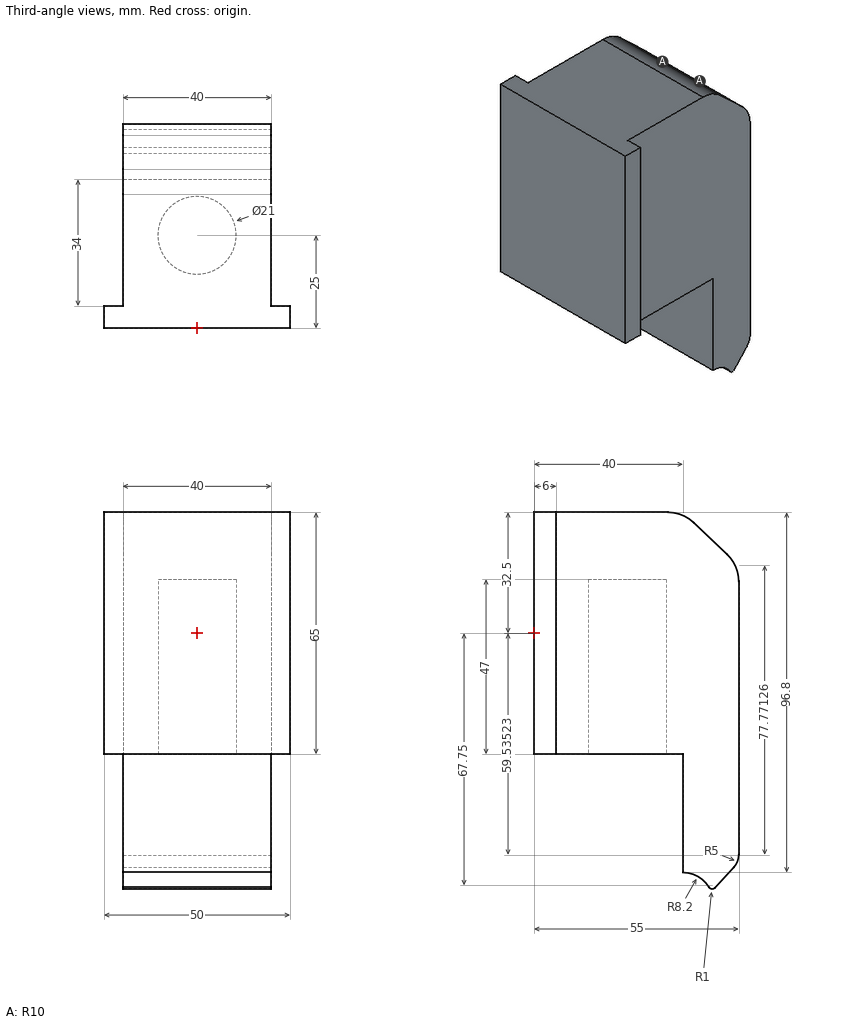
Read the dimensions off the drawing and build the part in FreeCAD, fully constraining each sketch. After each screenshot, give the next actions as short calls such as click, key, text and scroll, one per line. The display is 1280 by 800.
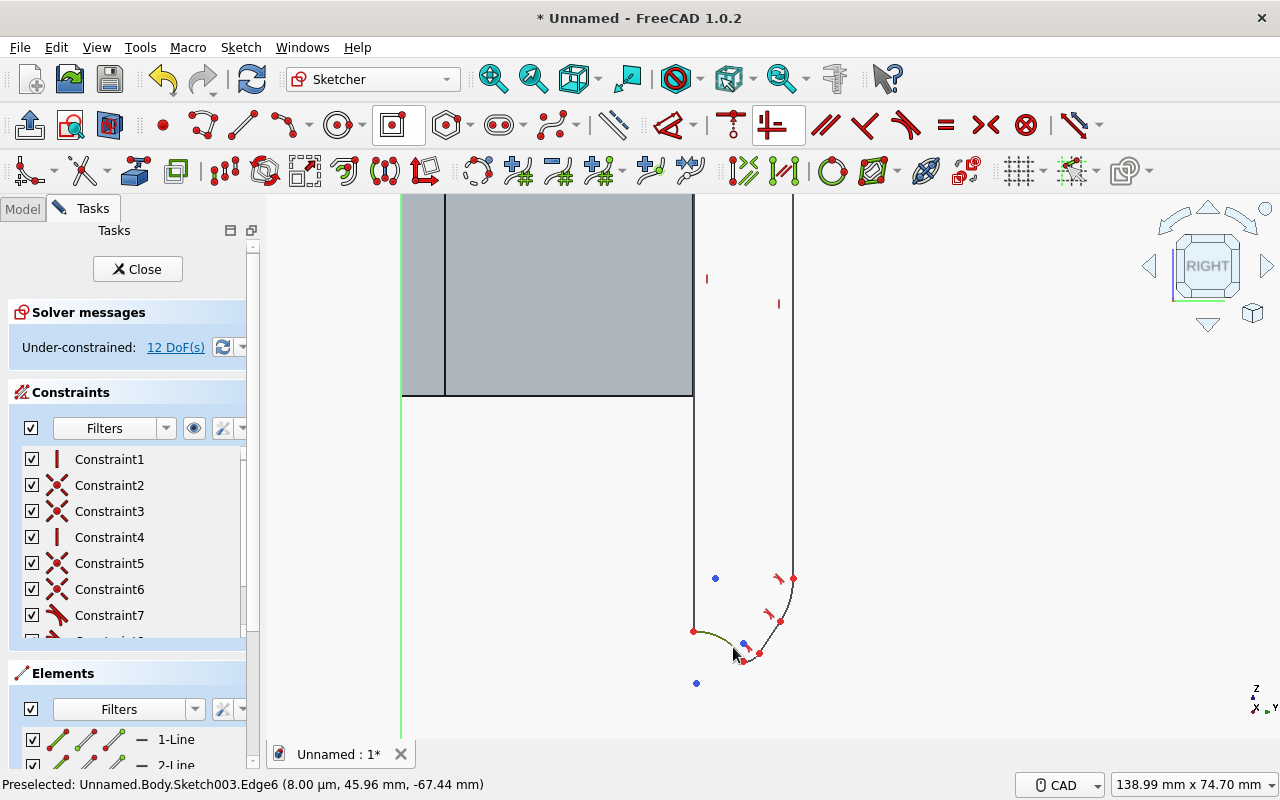
scroll(752, 660, up, 3)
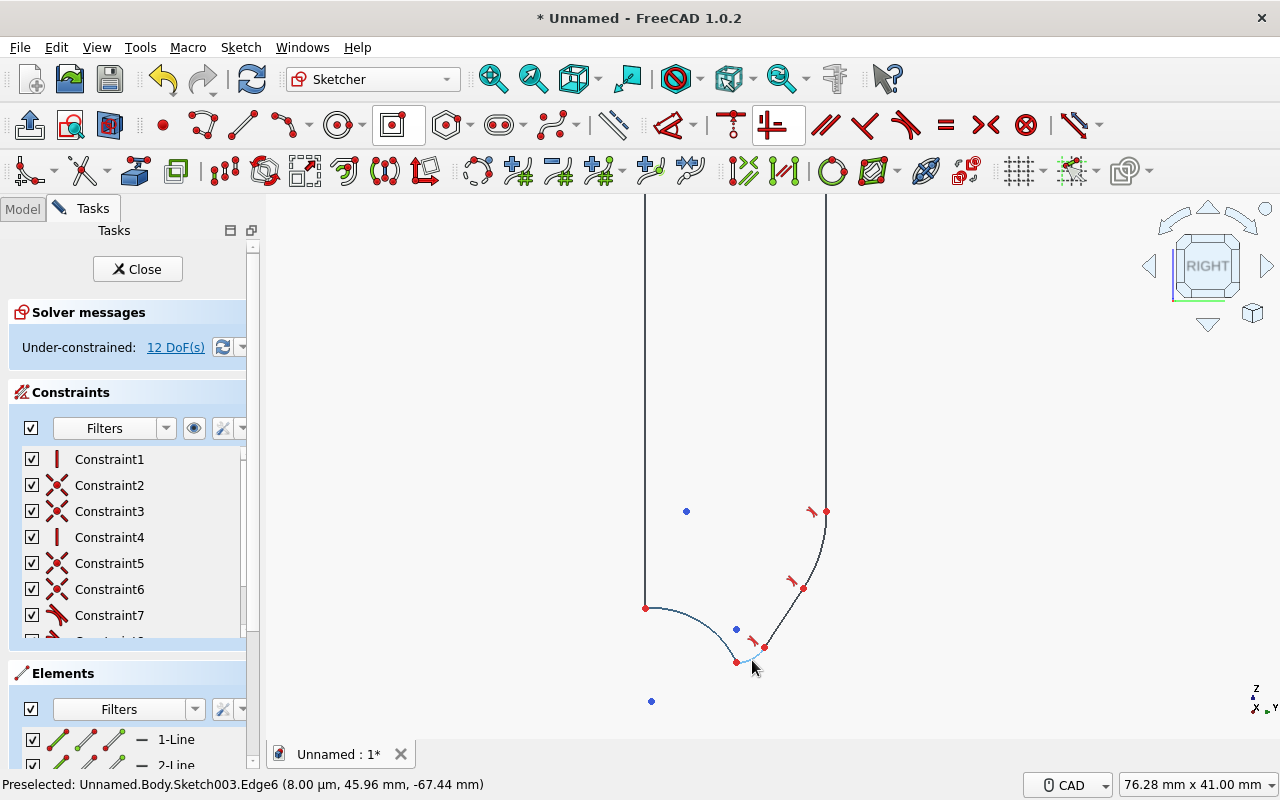
click(752, 659)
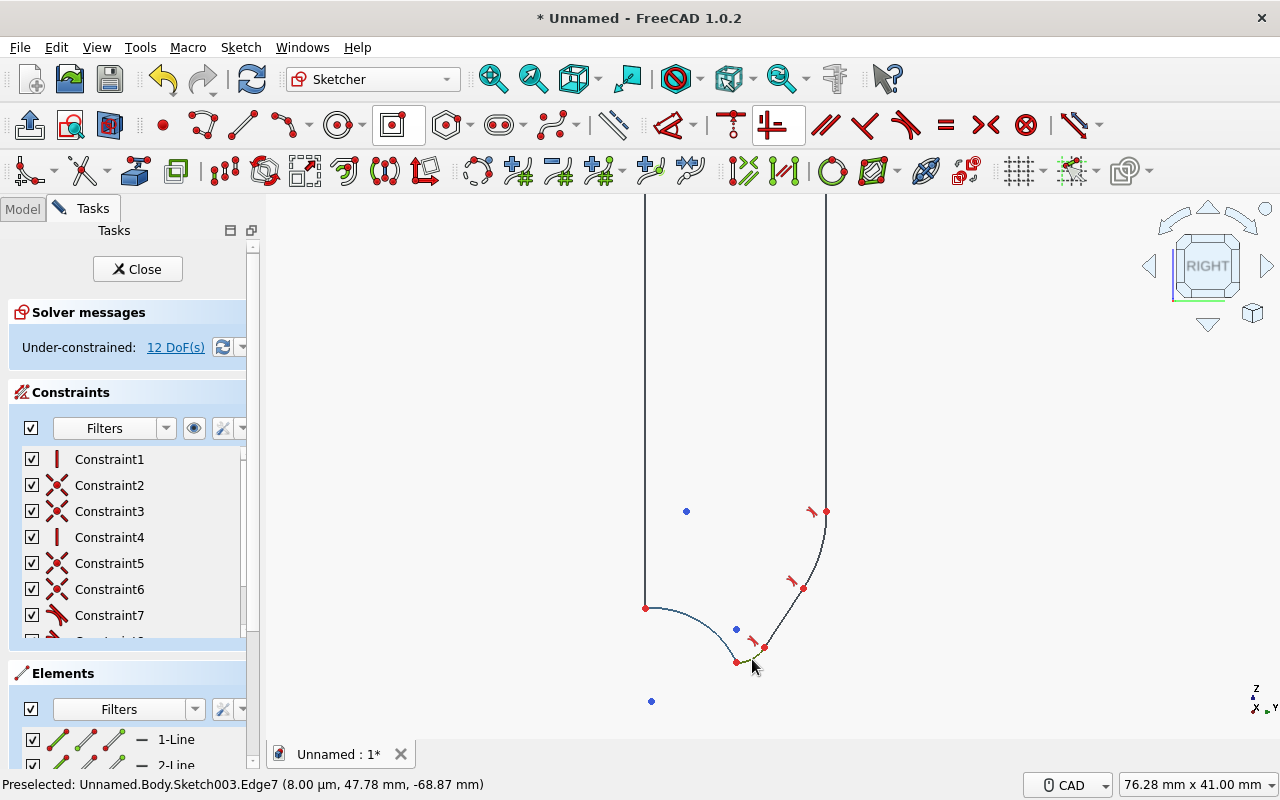
key(t)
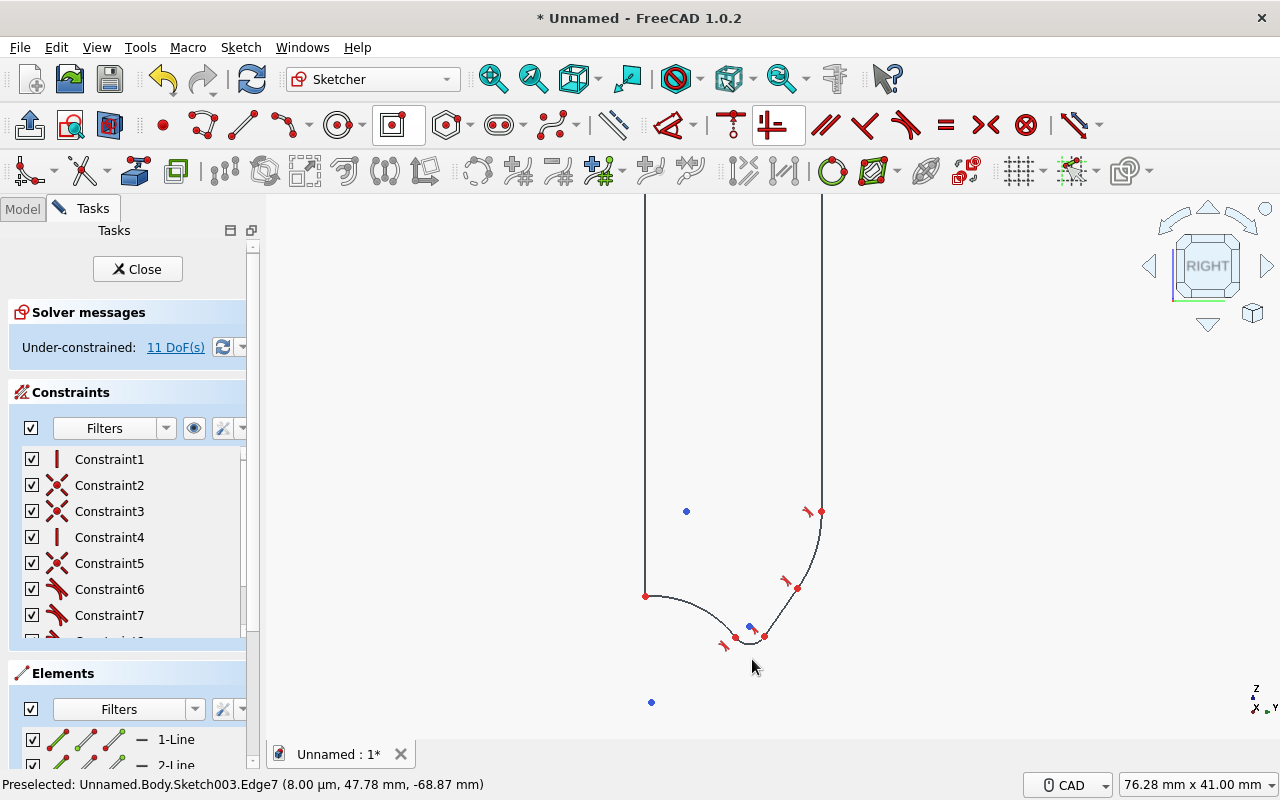
click(668, 126)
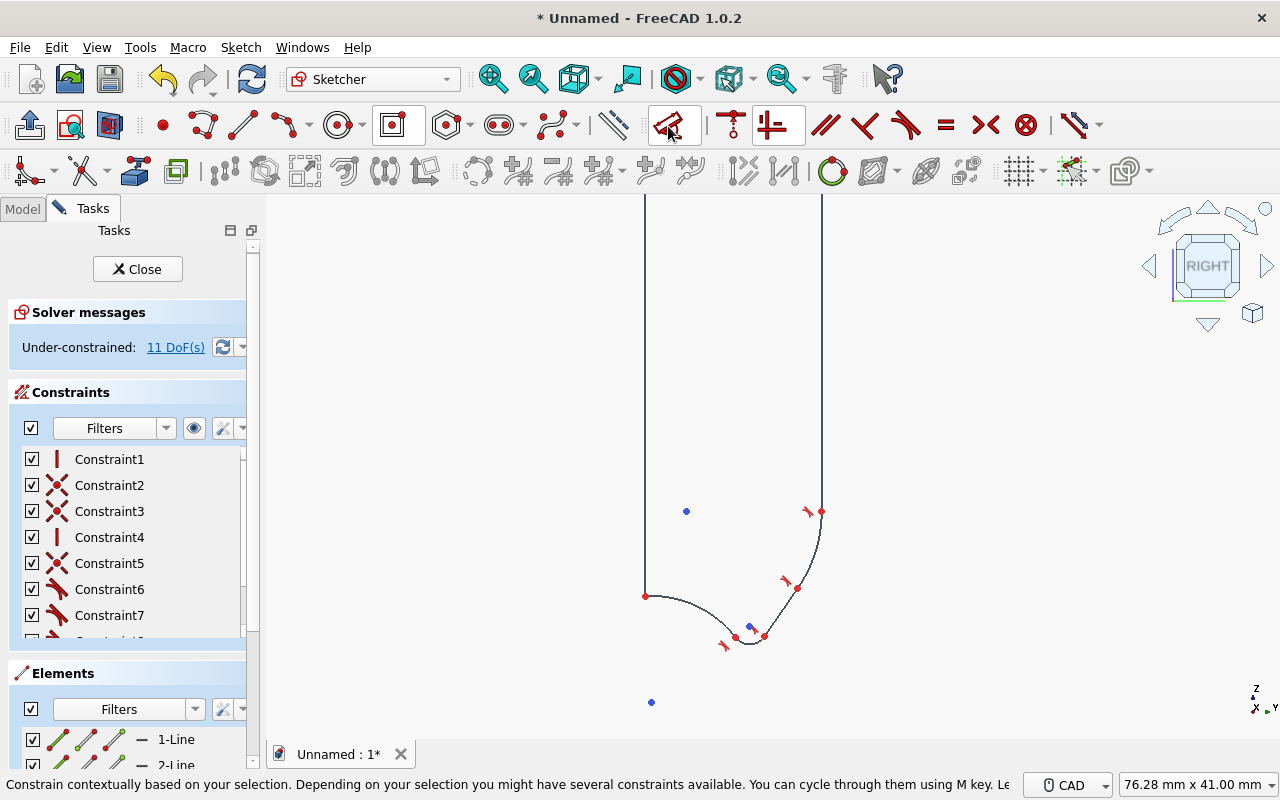
click(810, 567)
click(839, 580)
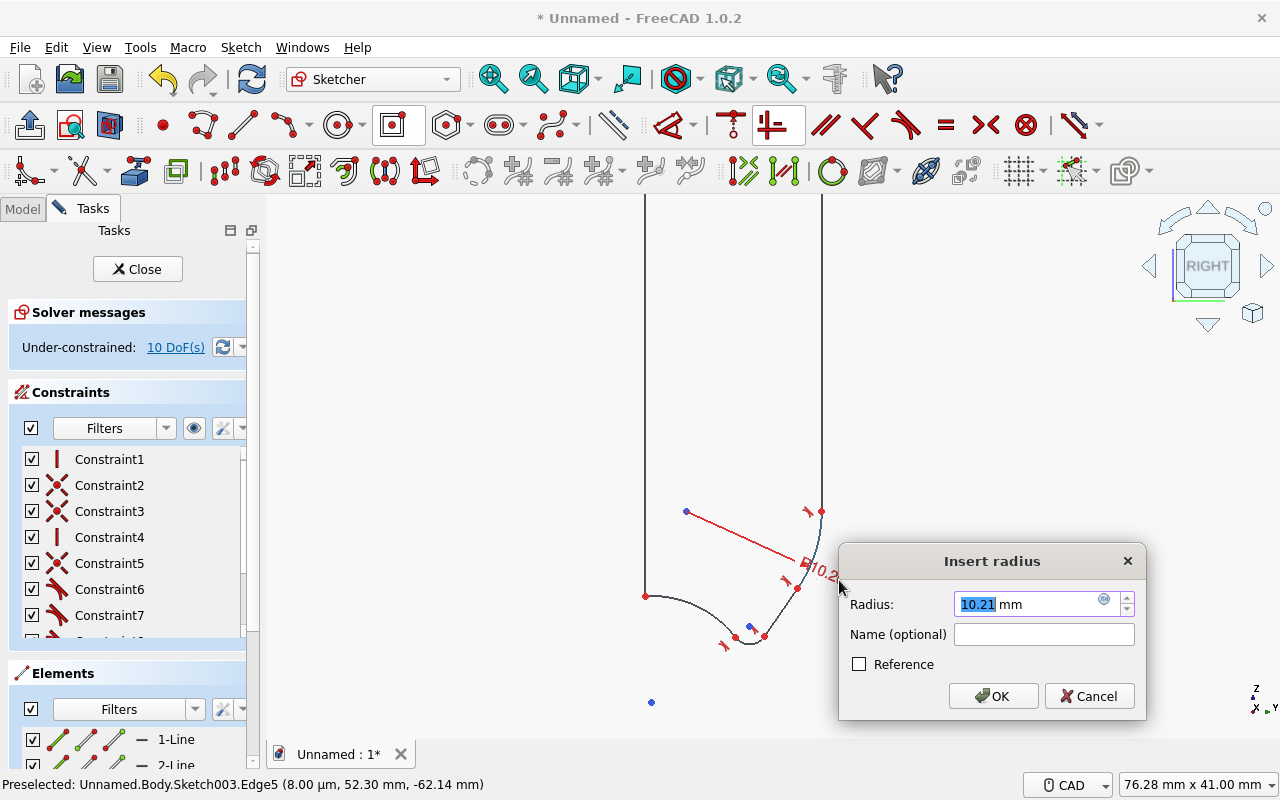
text(5)
key(Return)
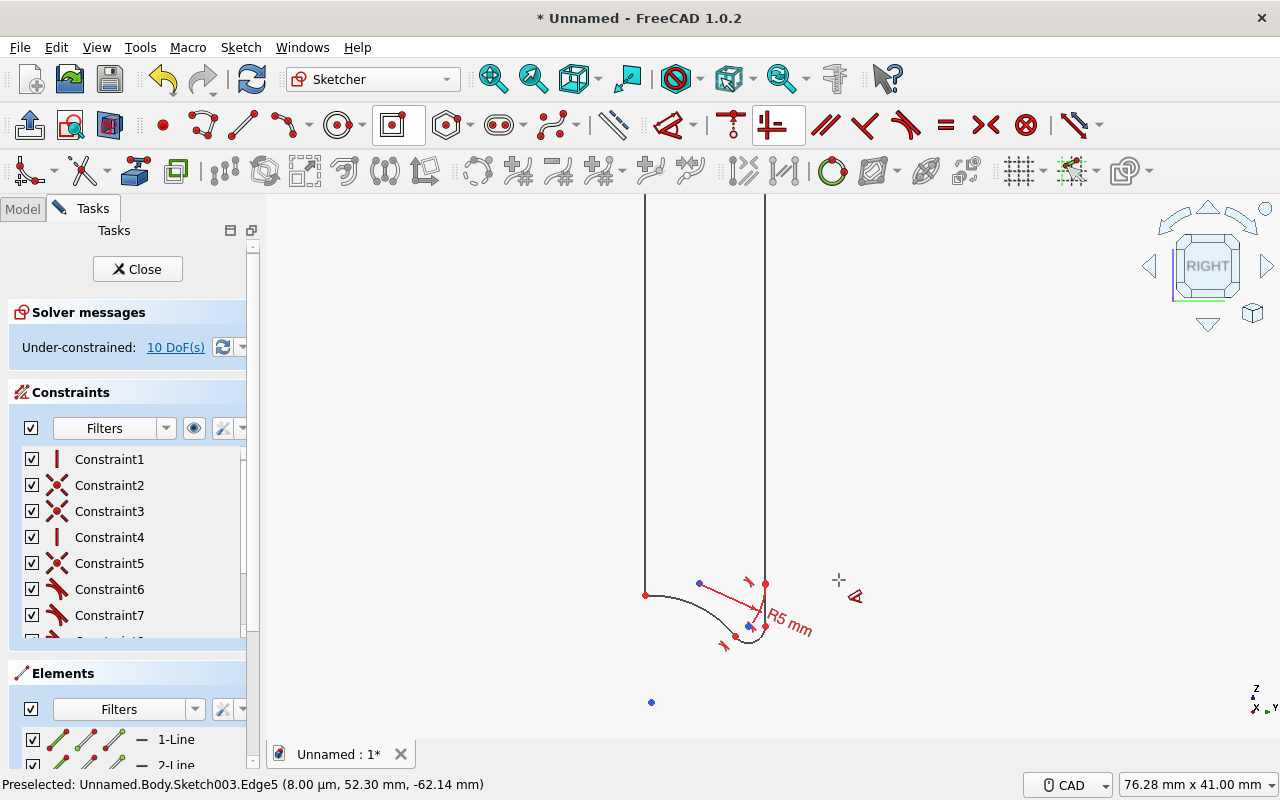
click(713, 615)
click(731, 589)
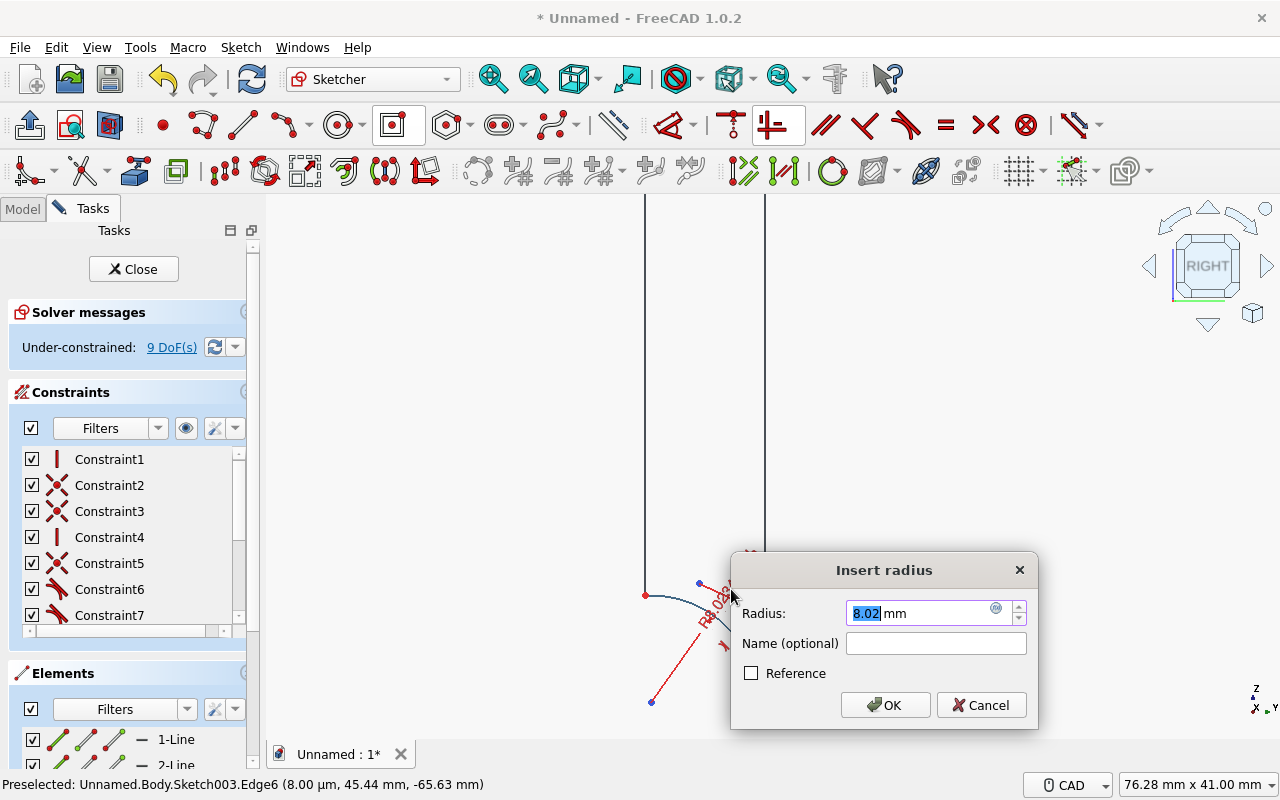
text(8.2)
key(Return)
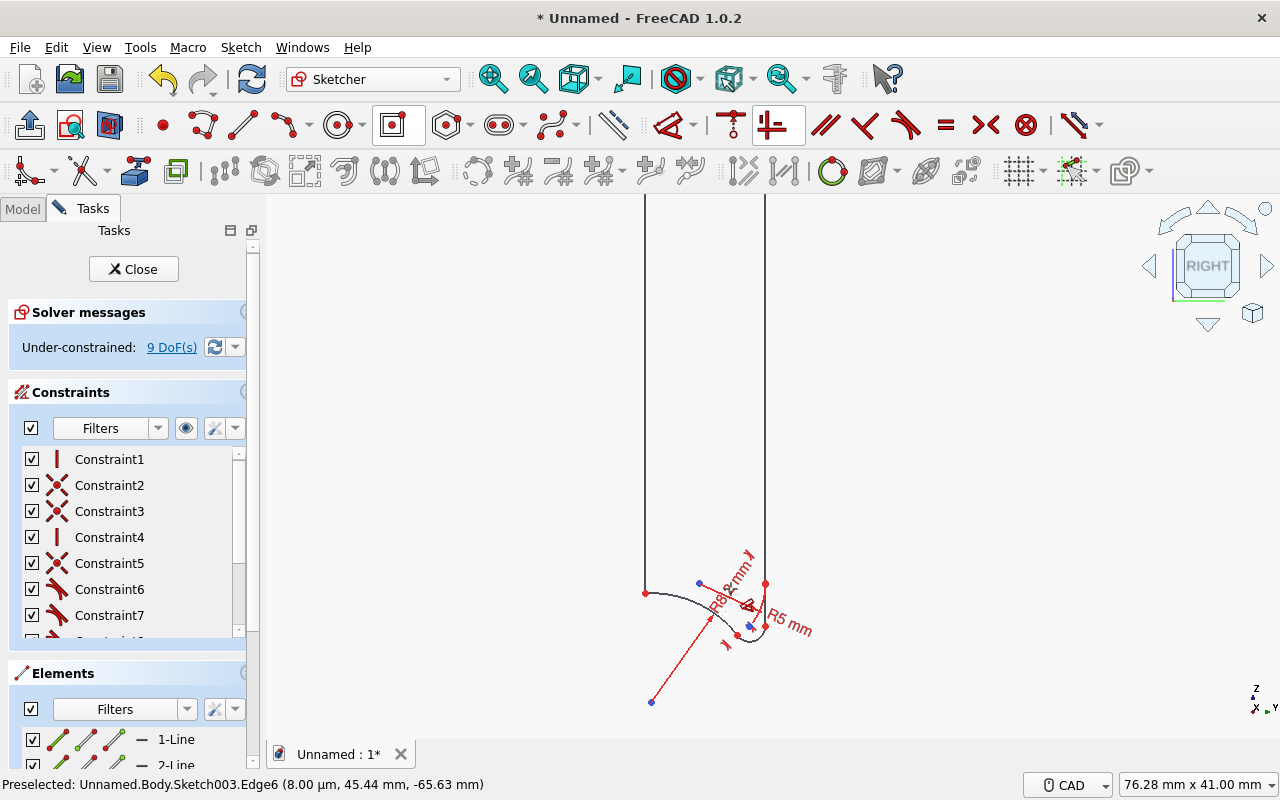
scroll(747, 642, up, 6)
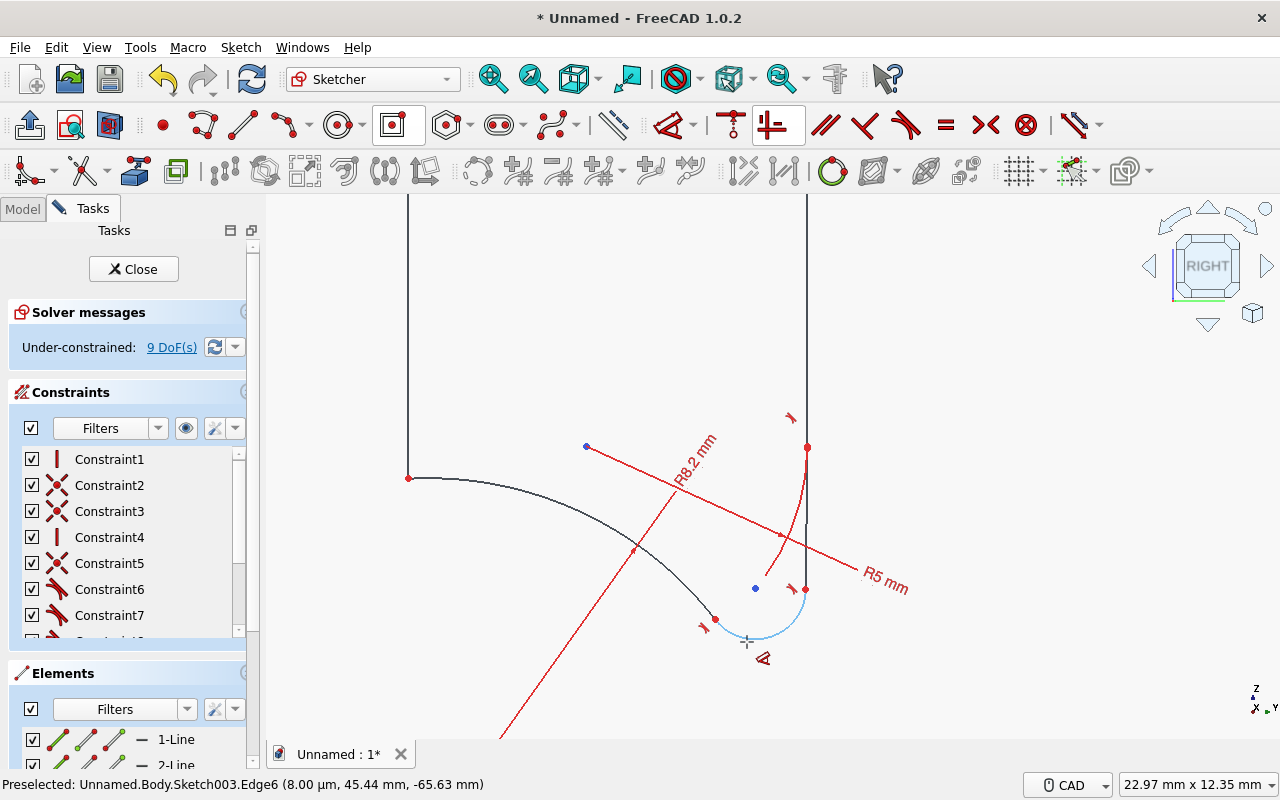
click(746, 638)
click(740, 669)